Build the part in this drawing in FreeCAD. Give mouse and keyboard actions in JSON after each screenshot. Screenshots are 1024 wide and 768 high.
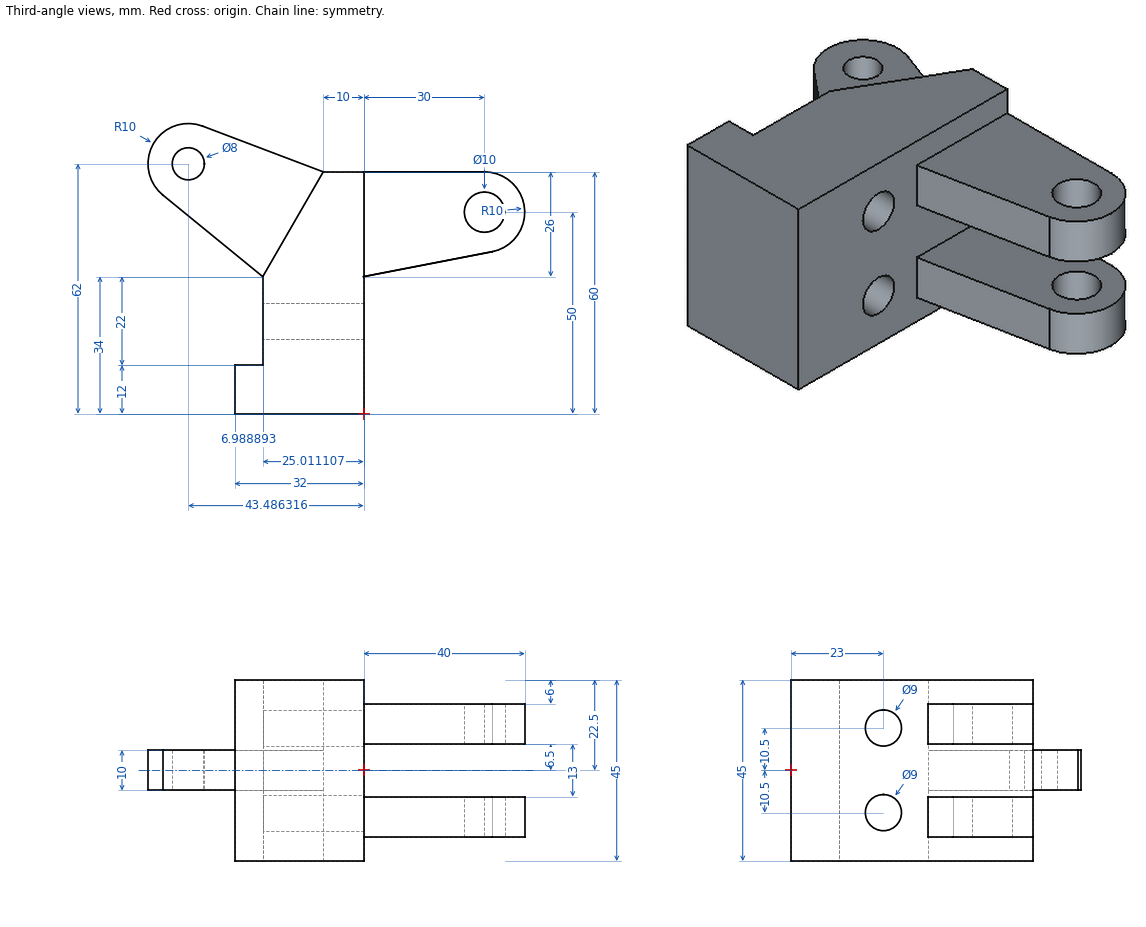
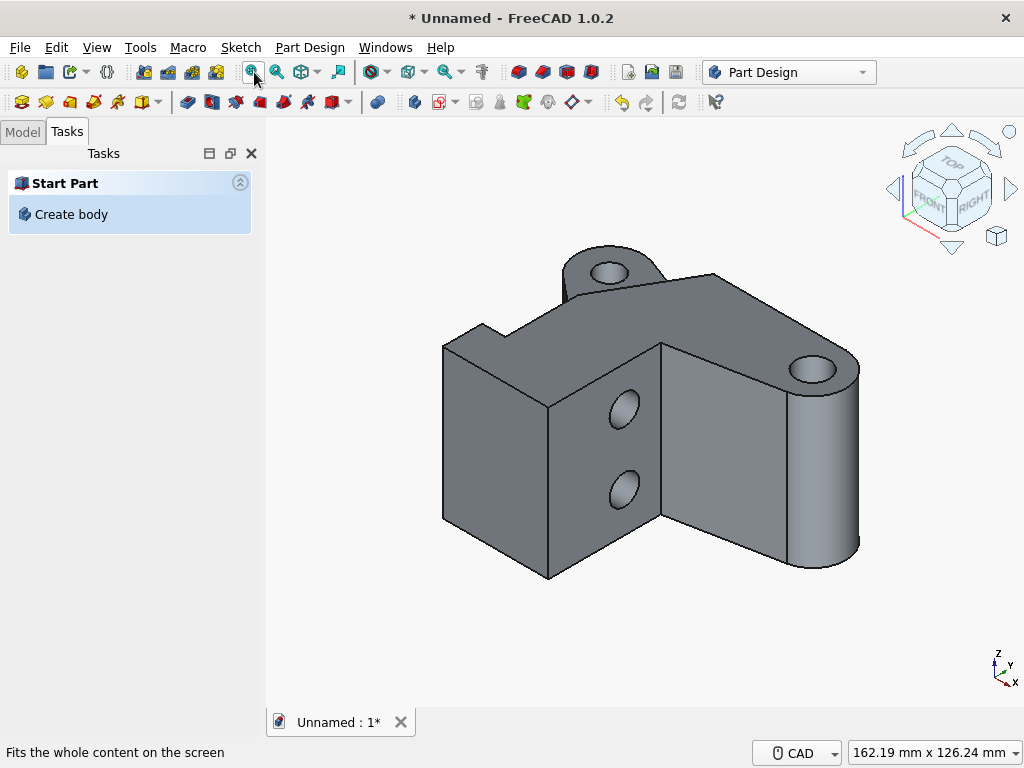
{"action": "key", "text": "4"}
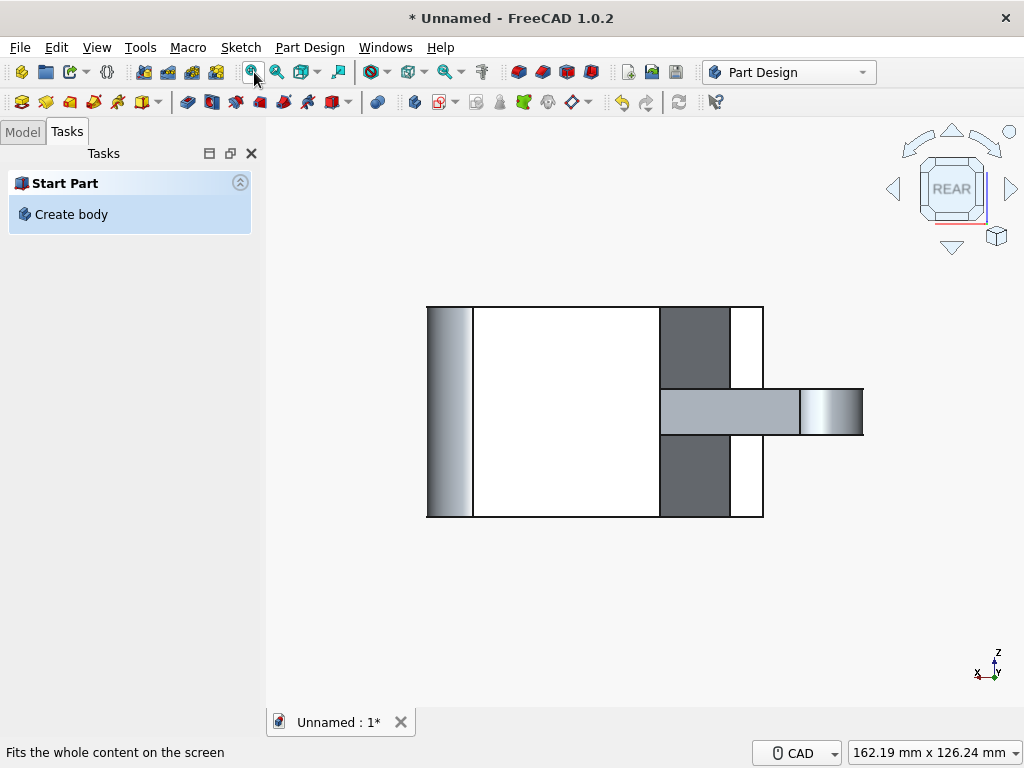
{"action": "left_click", "coordinate": [567, 411]}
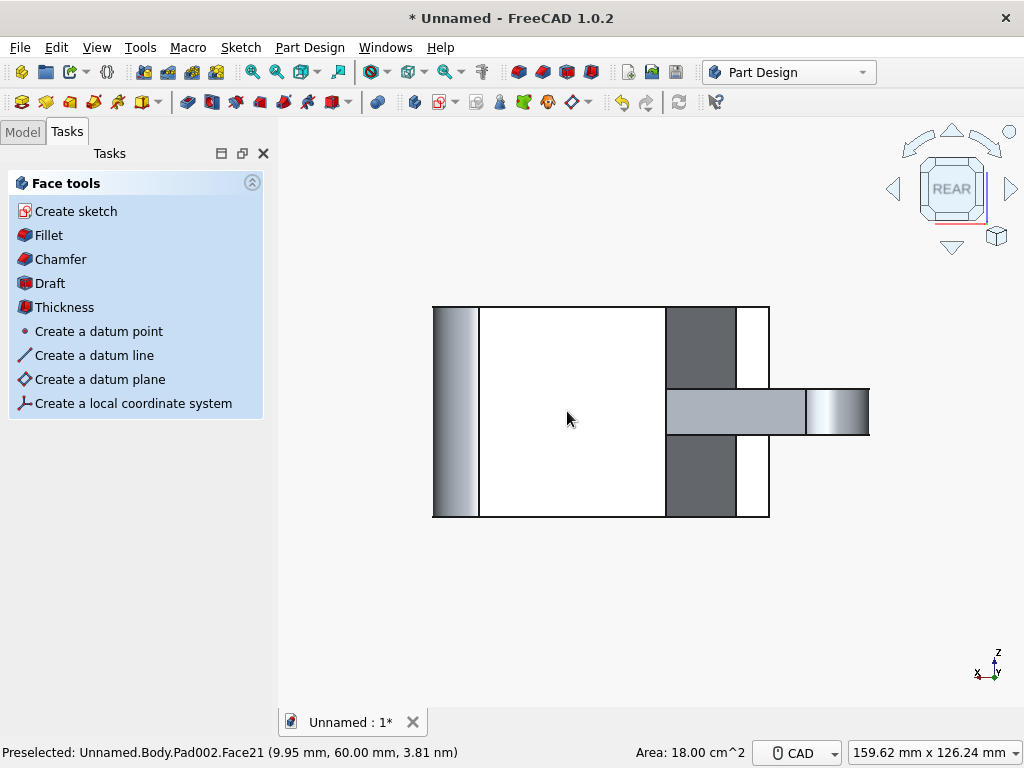
{"action": "left_click", "coordinate": [440, 102]}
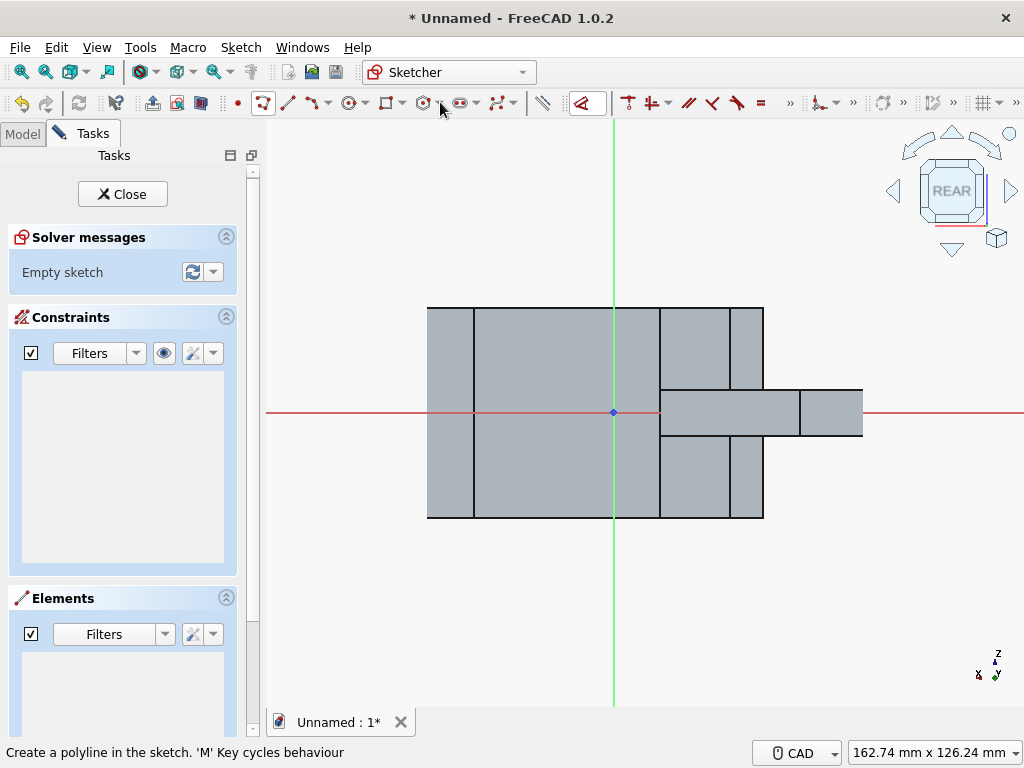
{"action": "key", "text": "q s"}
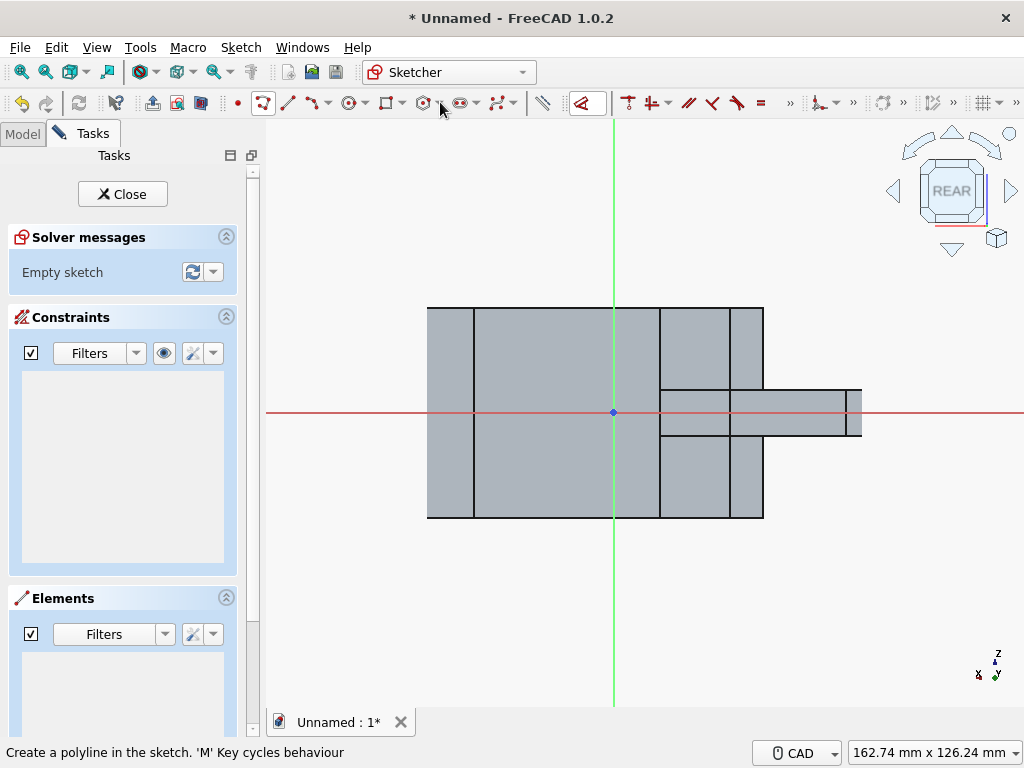
{"action": "scroll", "coordinate": [452, 413], "scroll_direction": "up", "scroll_amount": 3}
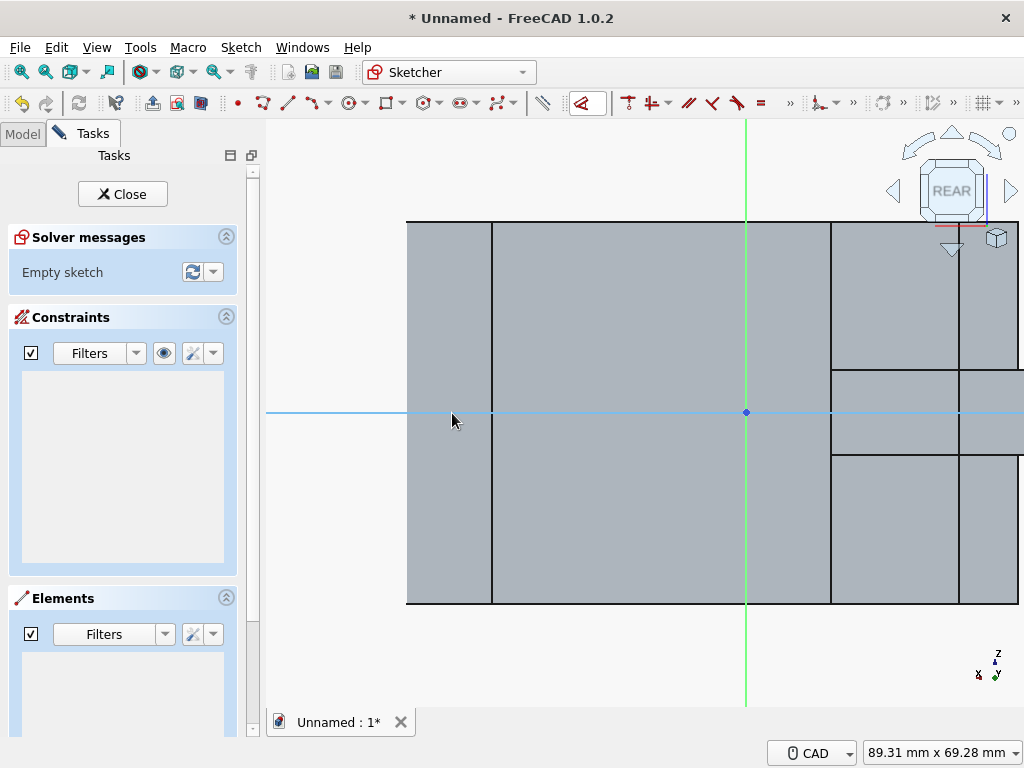
{"action": "key", "text": "g r"}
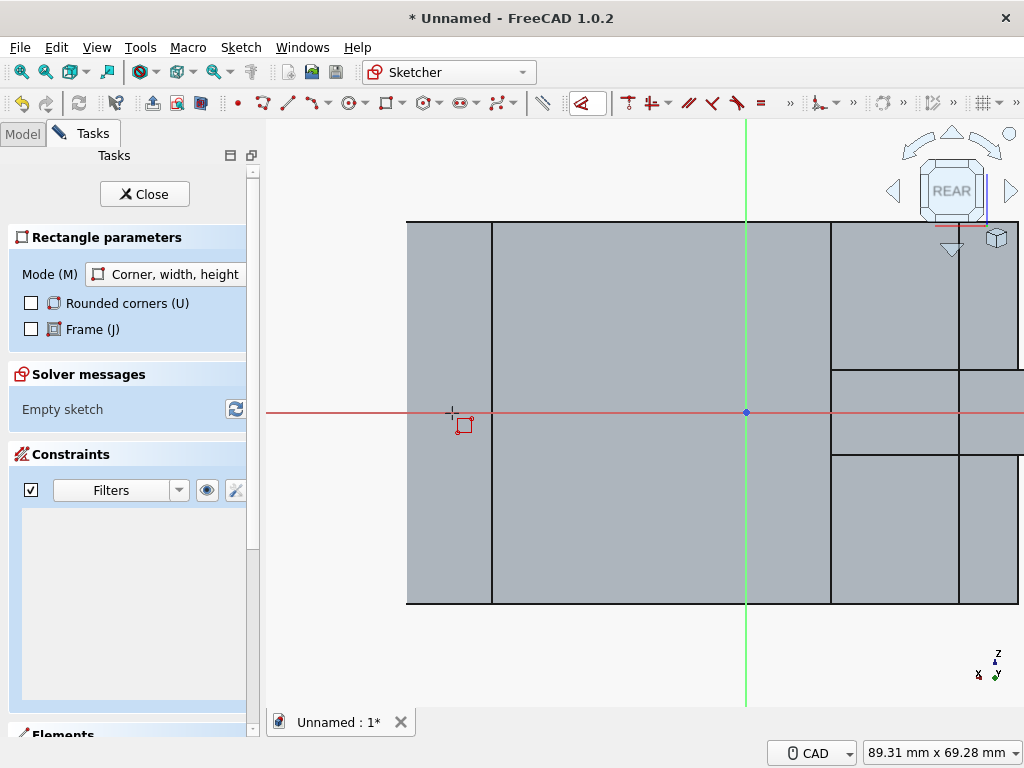
{"action": "left_click", "coordinate": [407, 222]}
{"action": "left_click", "coordinate": [746, 273]}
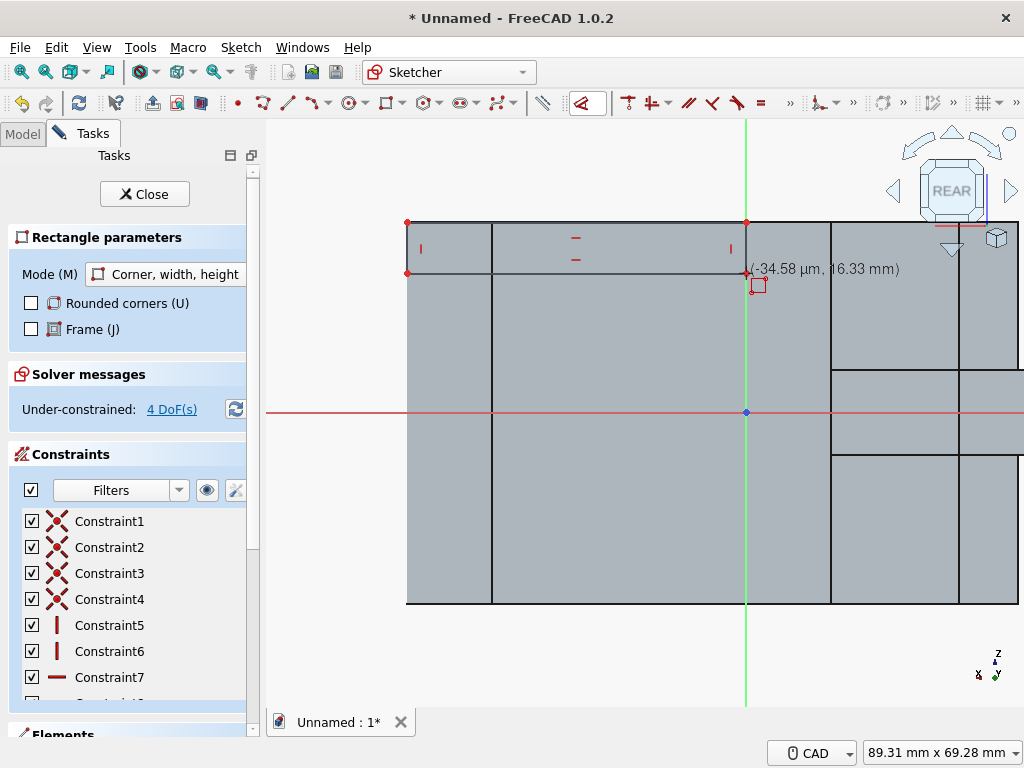
{"action": "left_click", "coordinate": [407, 357]}
{"action": "left_click", "coordinate": [746, 468]}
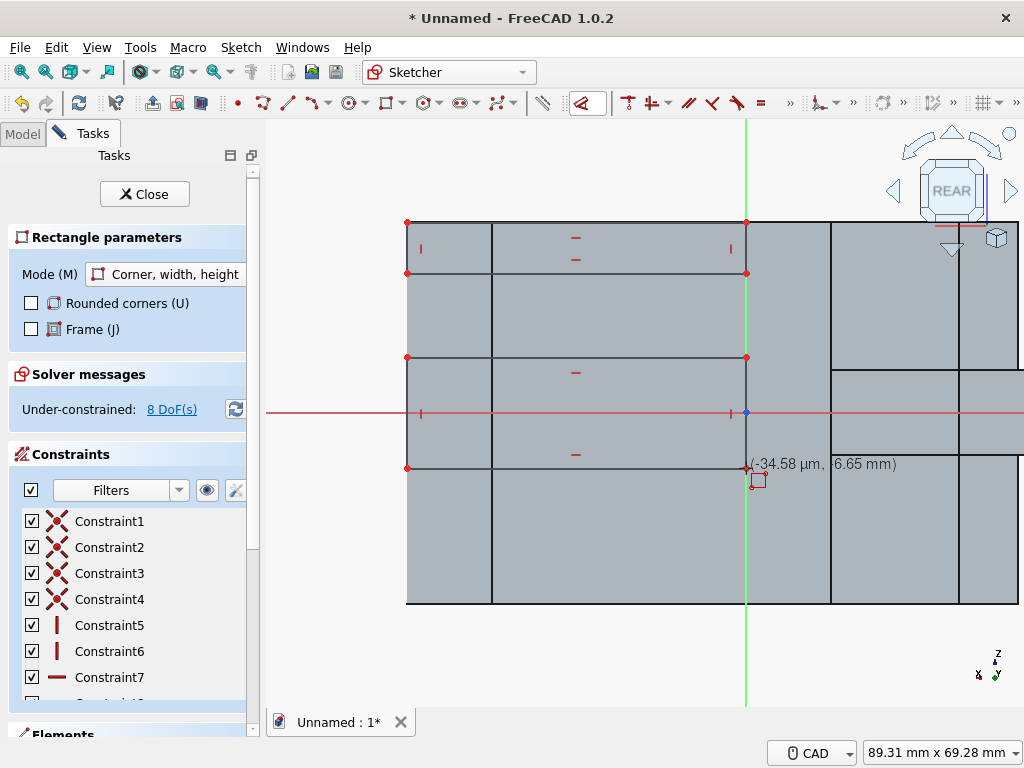
{"action": "left_click", "coordinate": [407, 553]}
{"action": "left_click", "coordinate": [746, 604]}
{"action": "key", "text": "Escape"}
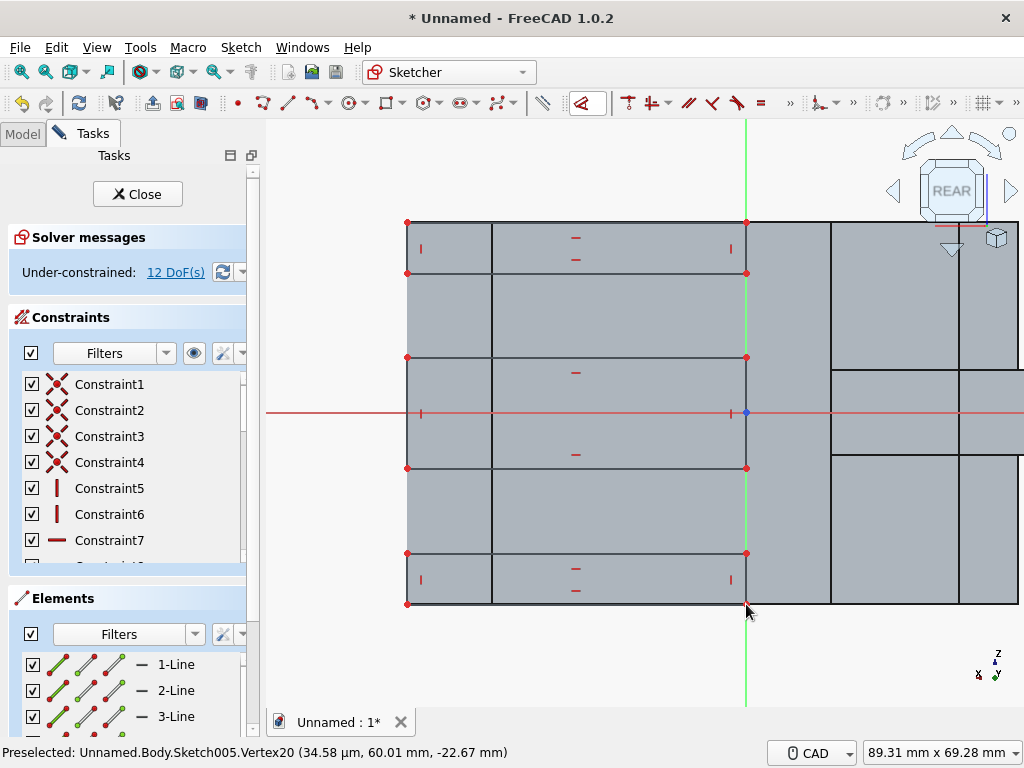
{"action": "left_click", "coordinate": [407, 274]}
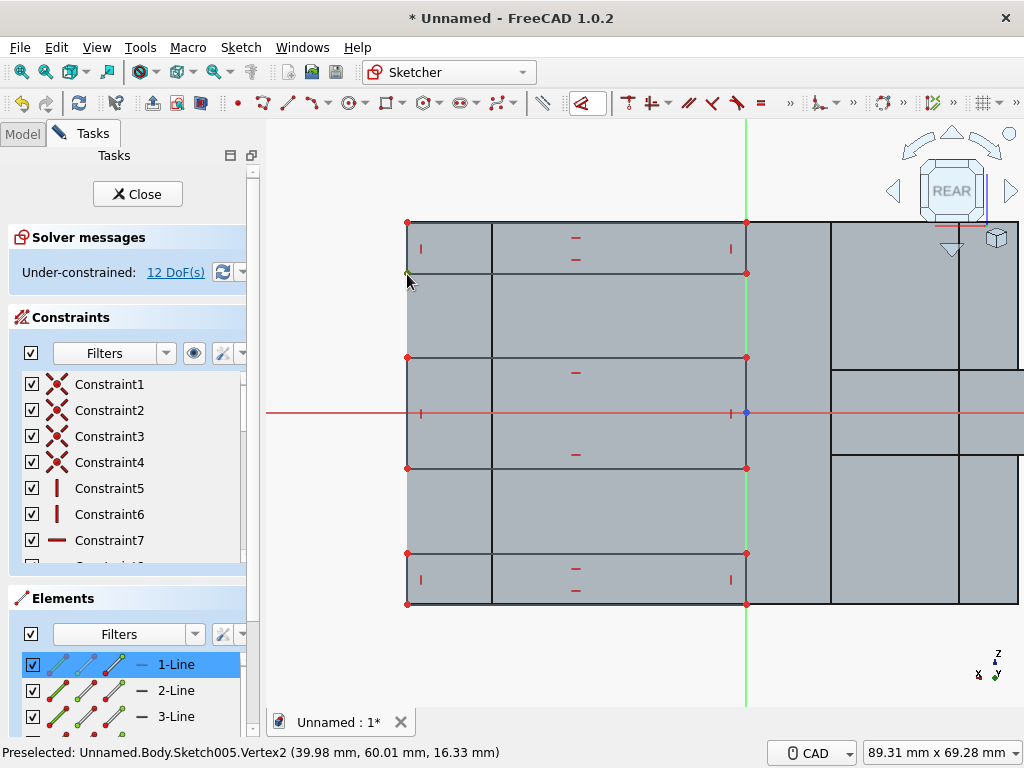
{"action": "left_click", "coordinate": [407, 554]}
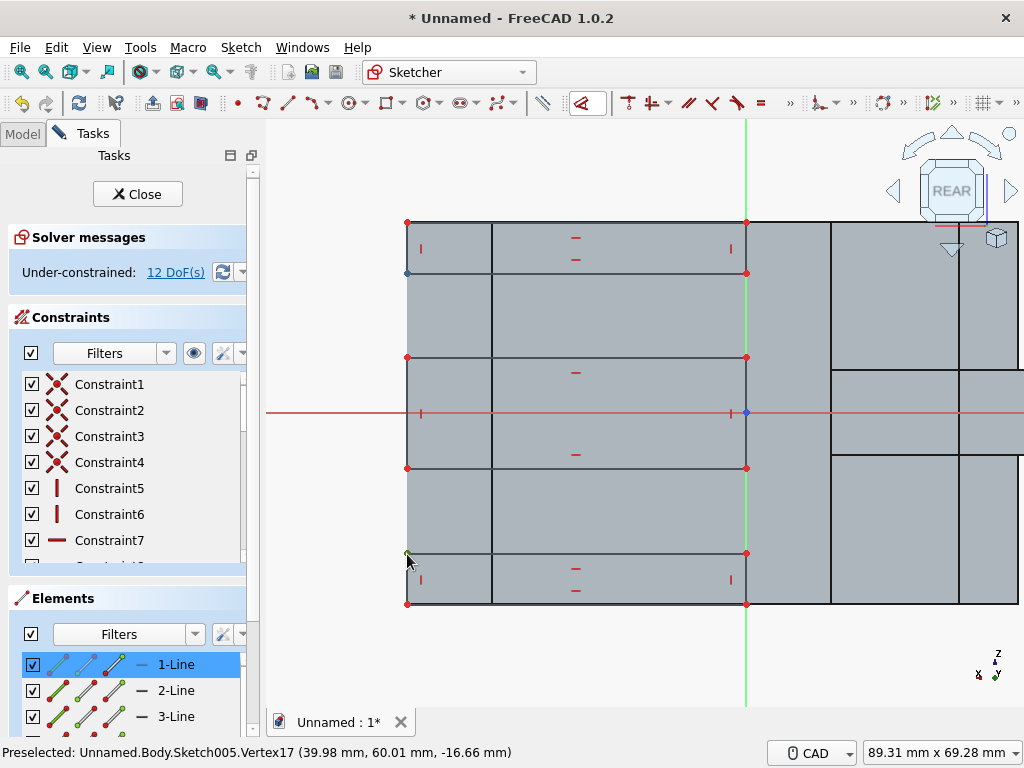
{"action": "left_click", "coordinate": [334, 413]}